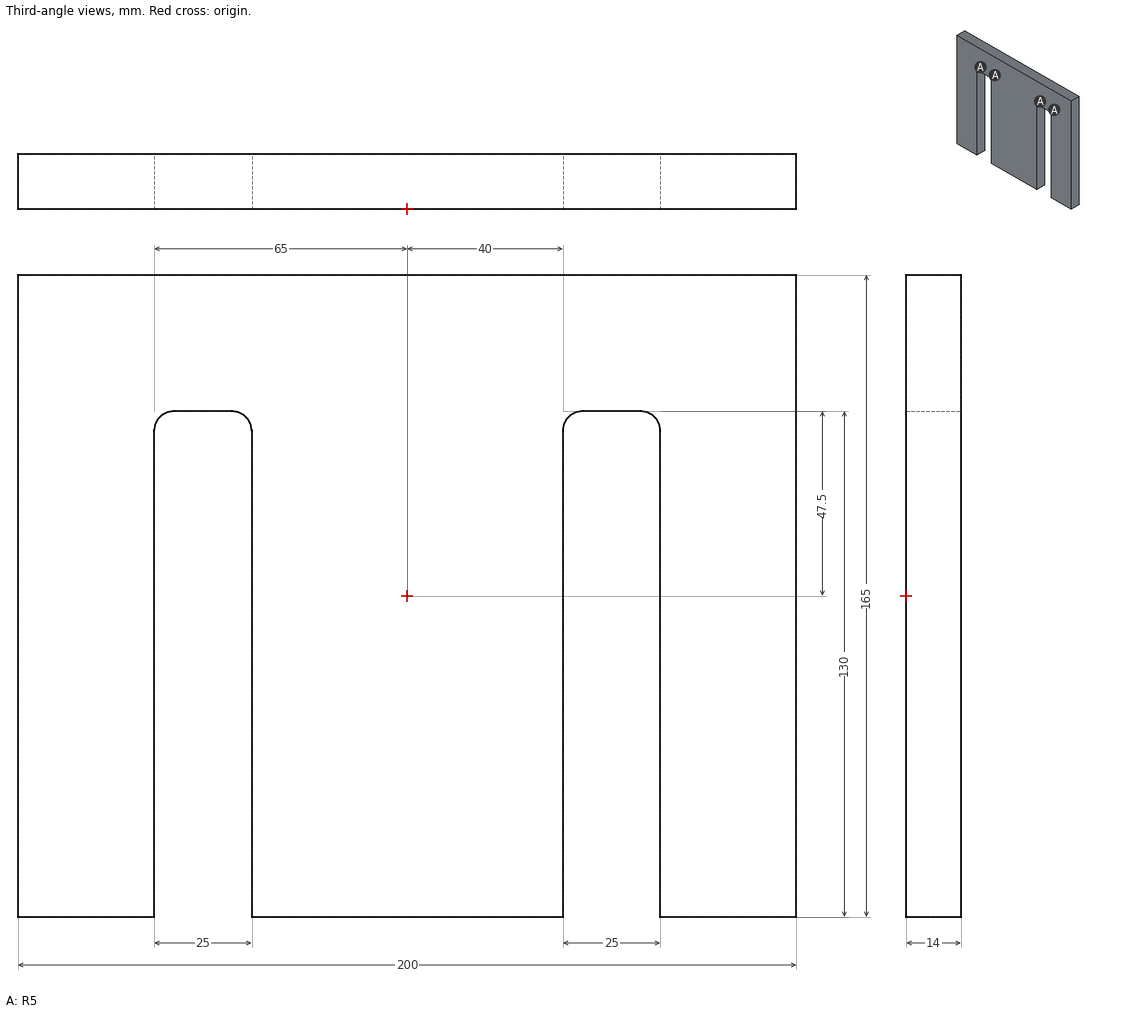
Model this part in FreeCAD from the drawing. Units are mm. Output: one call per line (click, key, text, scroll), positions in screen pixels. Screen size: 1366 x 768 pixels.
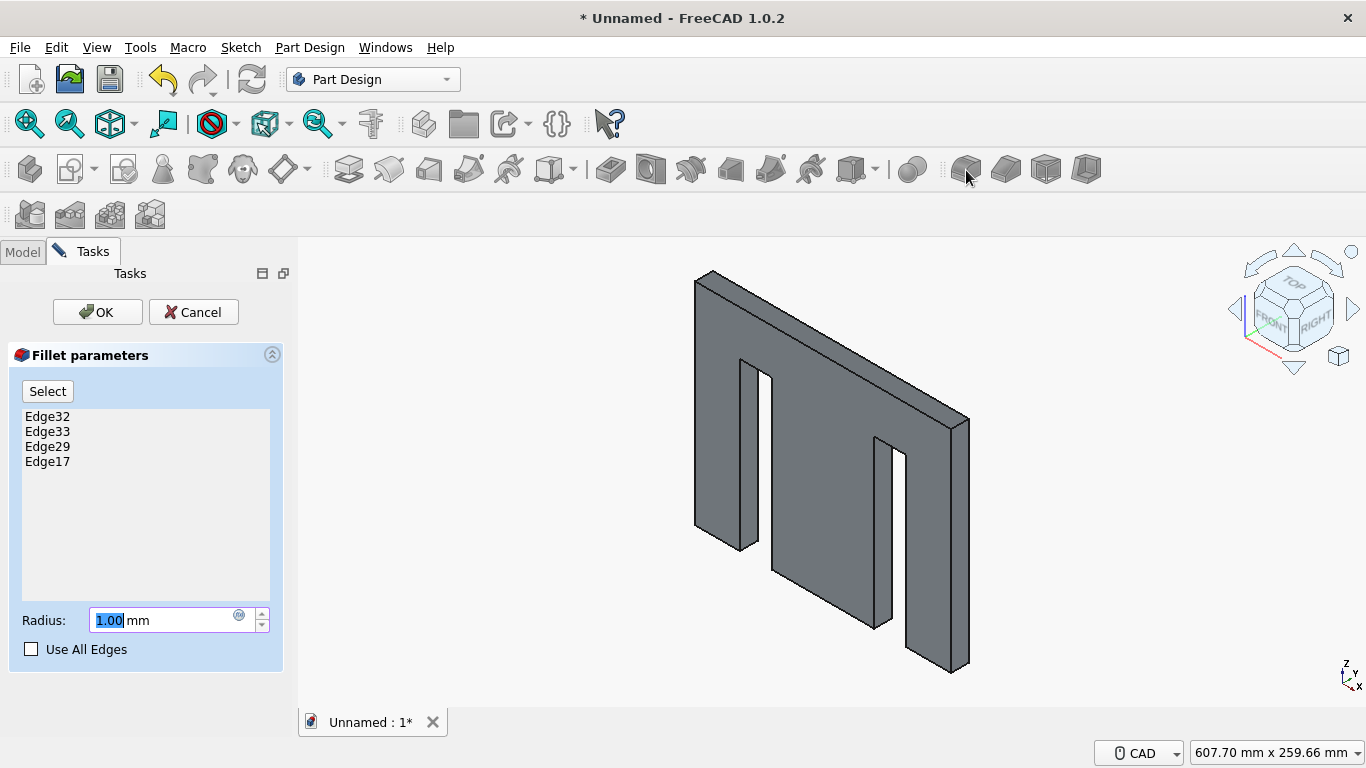
text(5)
key(Tab)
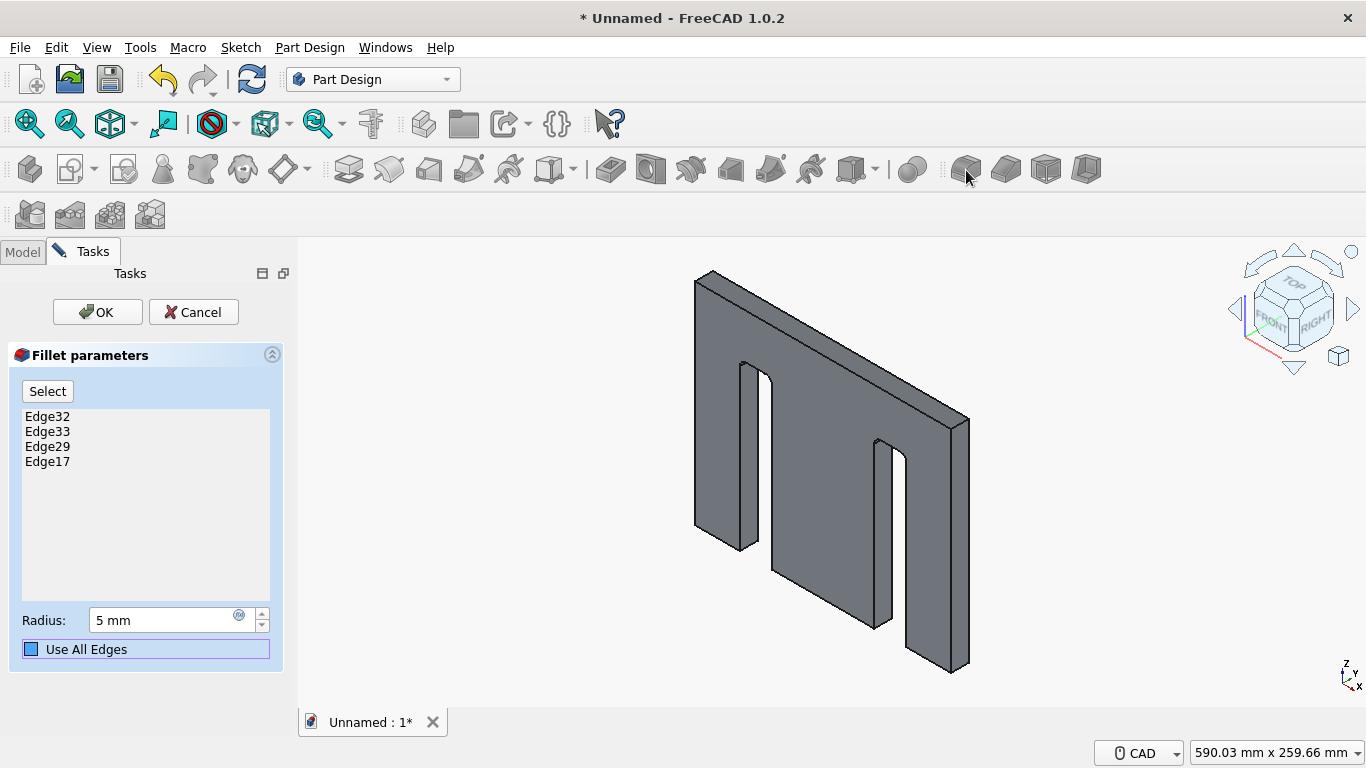
click(98, 312)